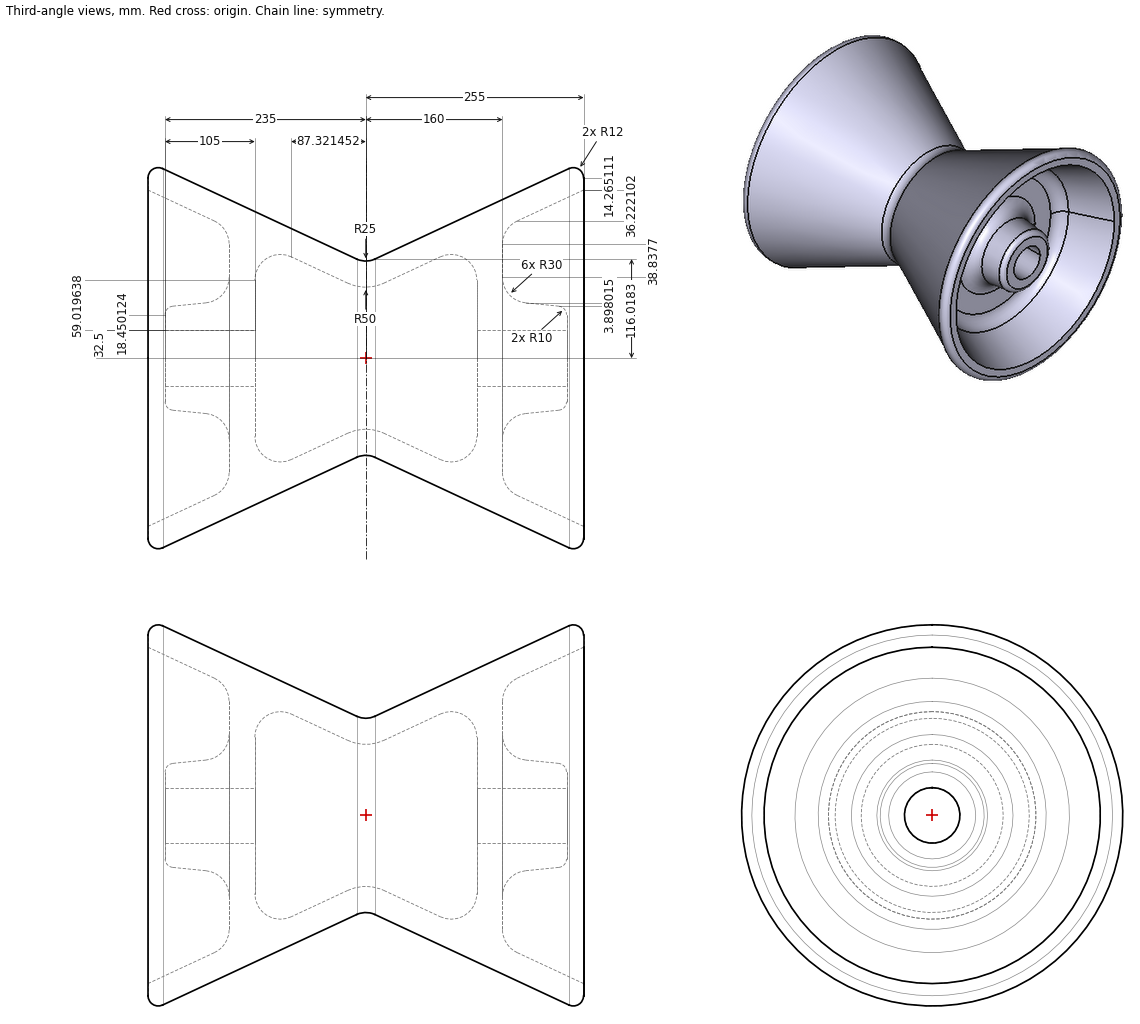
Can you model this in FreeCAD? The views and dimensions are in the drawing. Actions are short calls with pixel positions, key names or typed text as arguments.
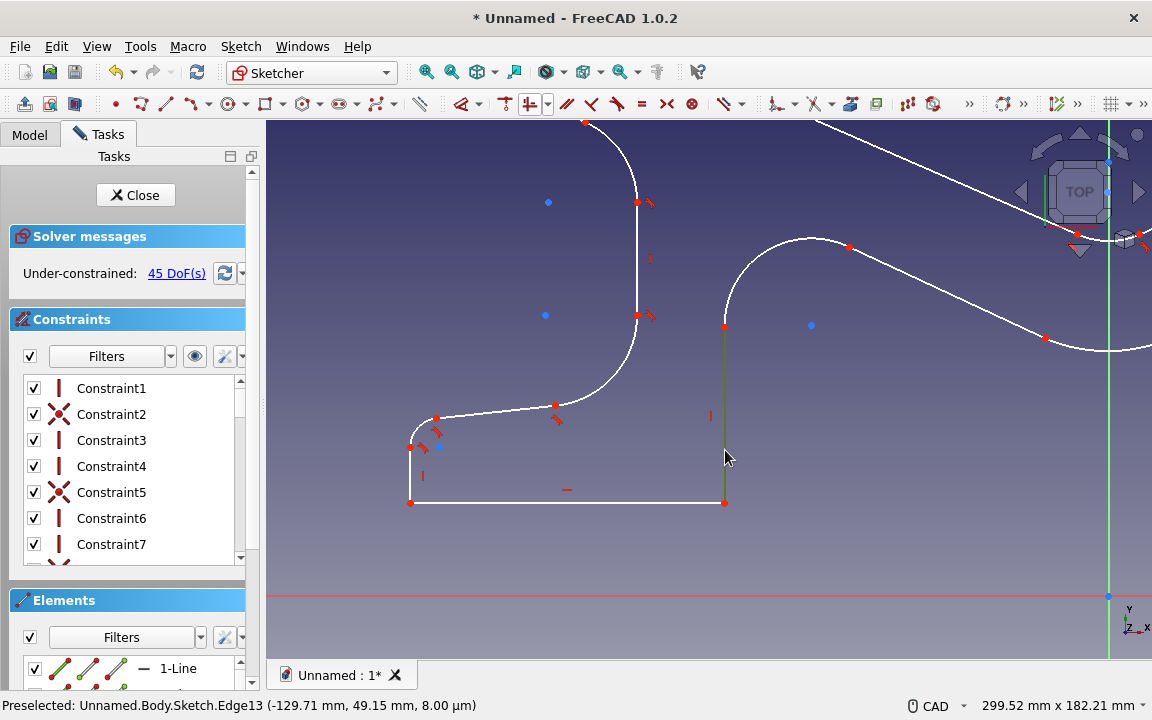
click(798, 240)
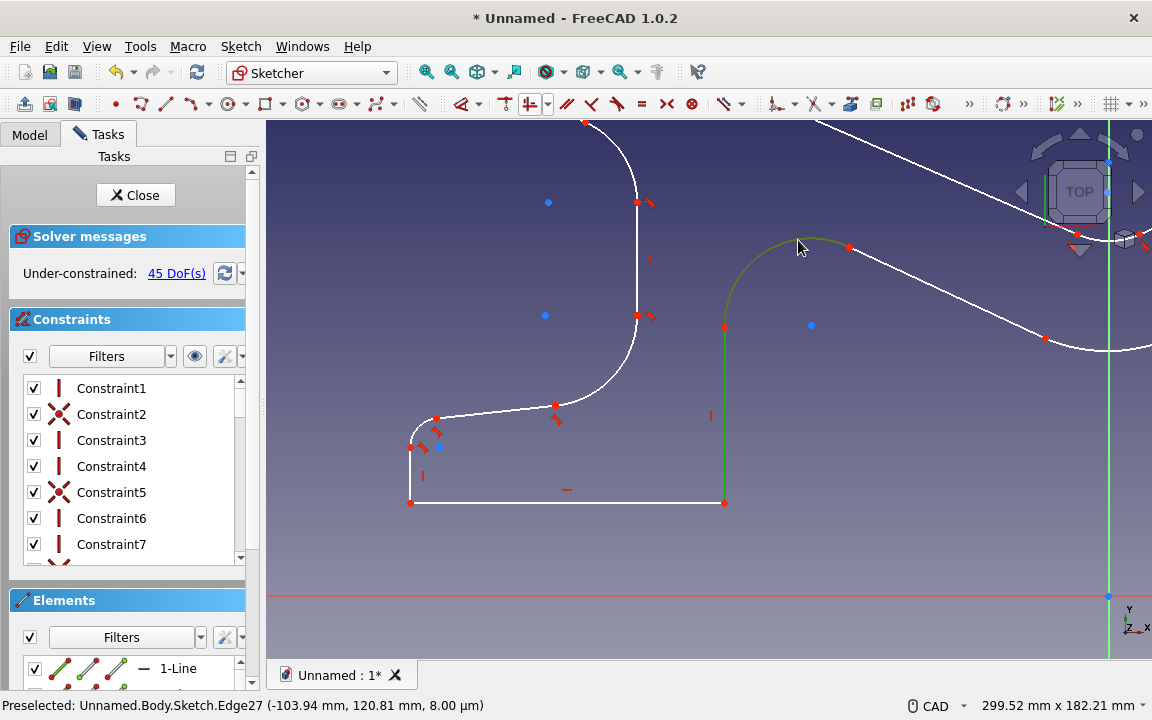
key(t)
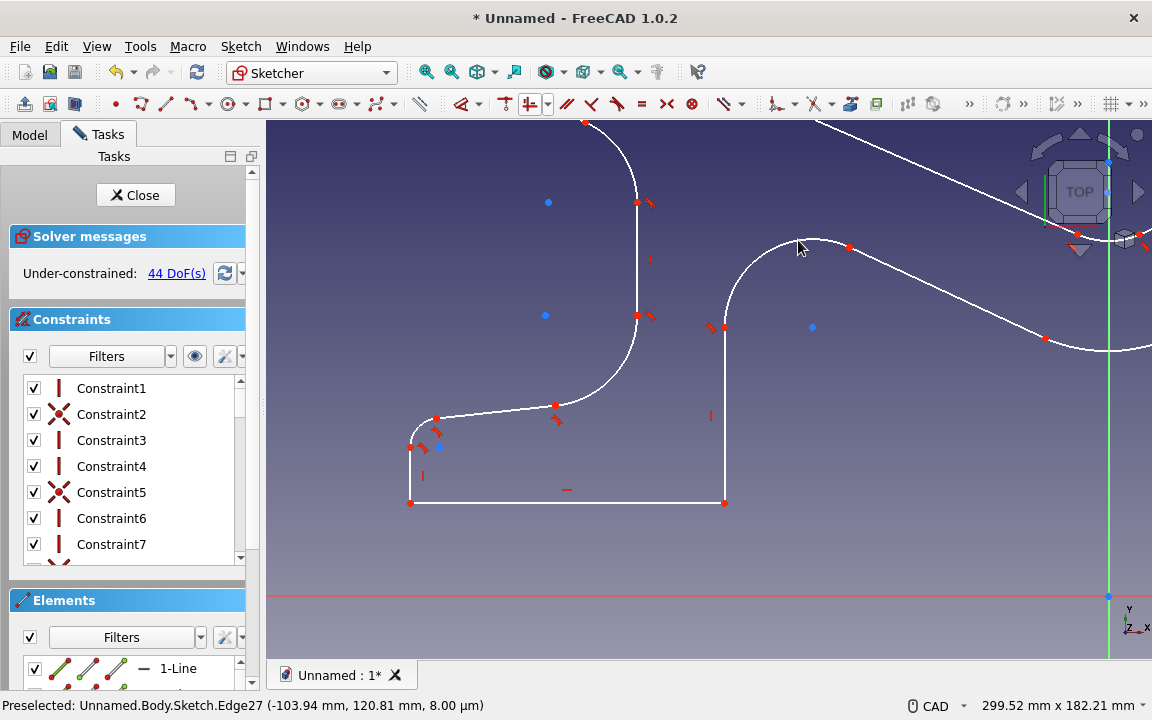
click(908, 275)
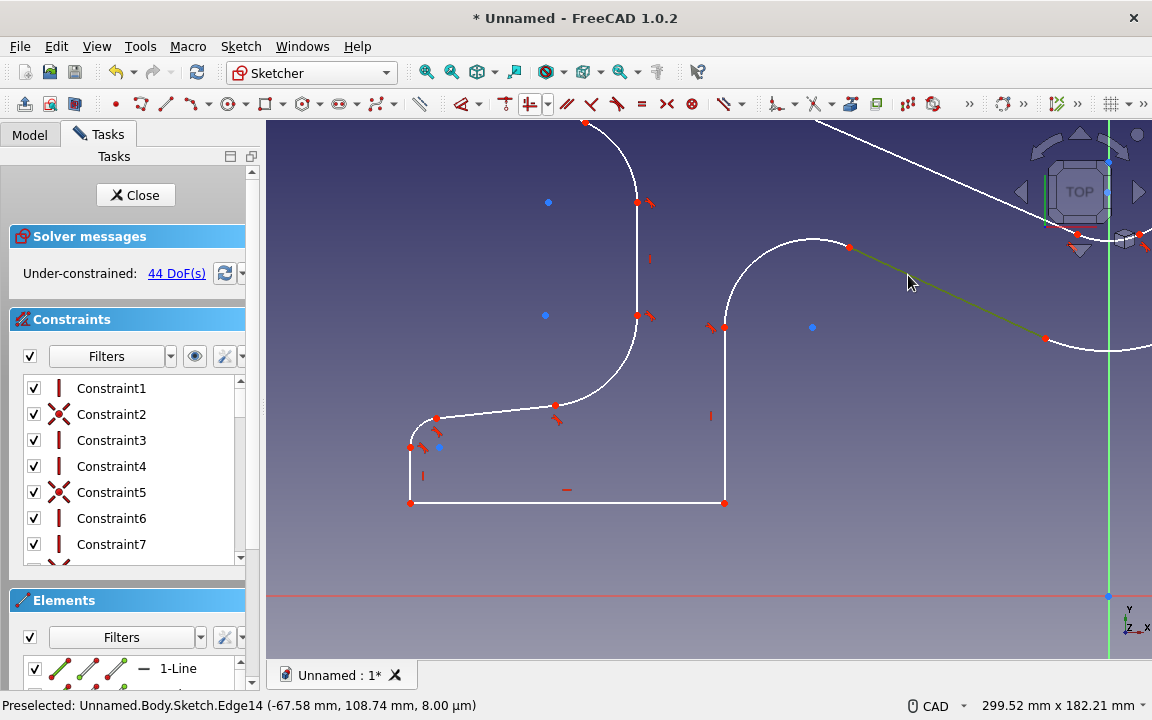
click(798, 241)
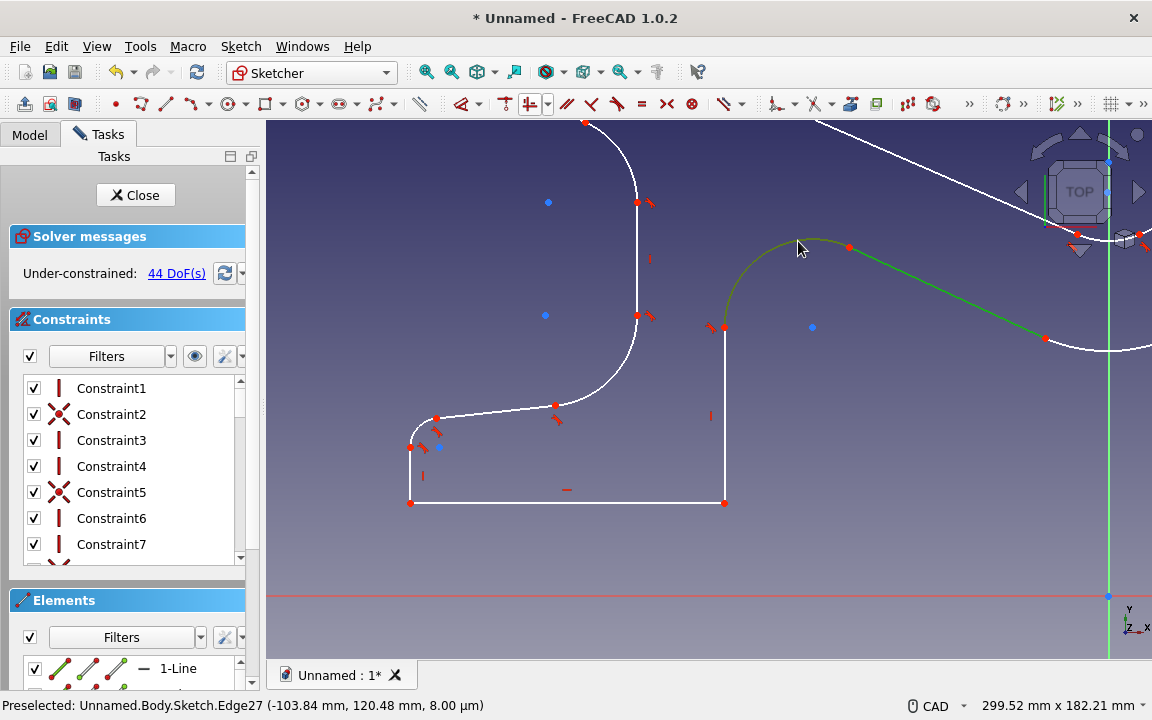
key(t)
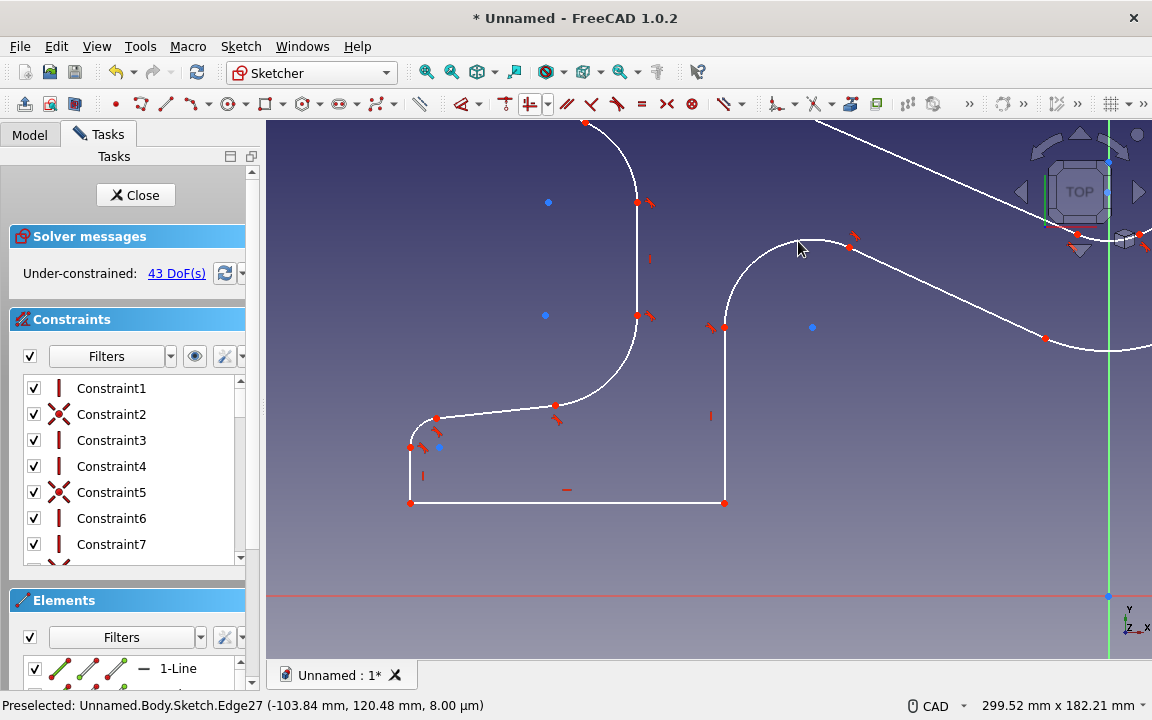
click(908, 275)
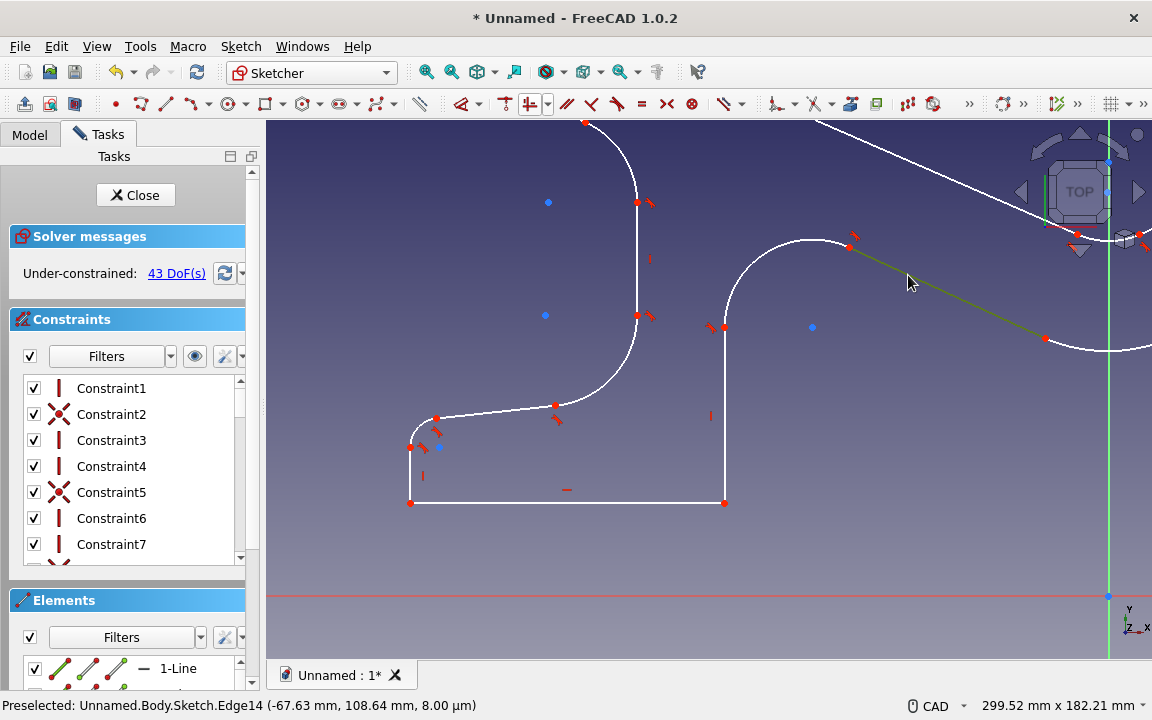
scroll(439, 442, down, 6)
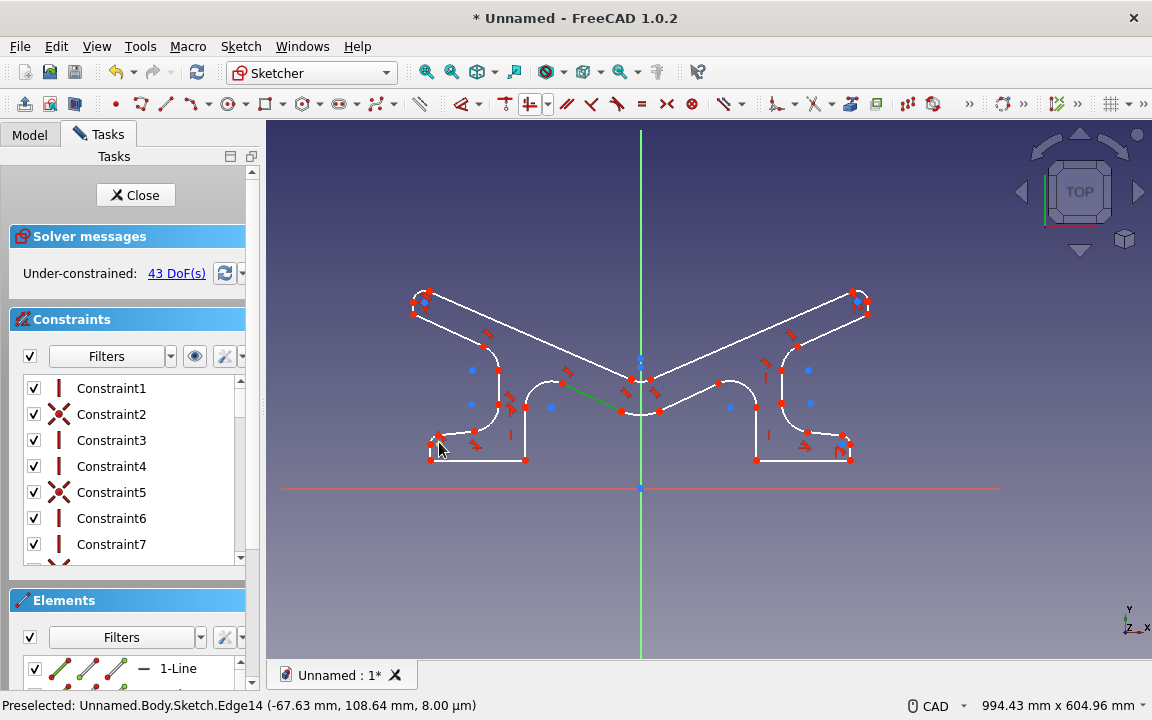
scroll(633, 414, up, 3)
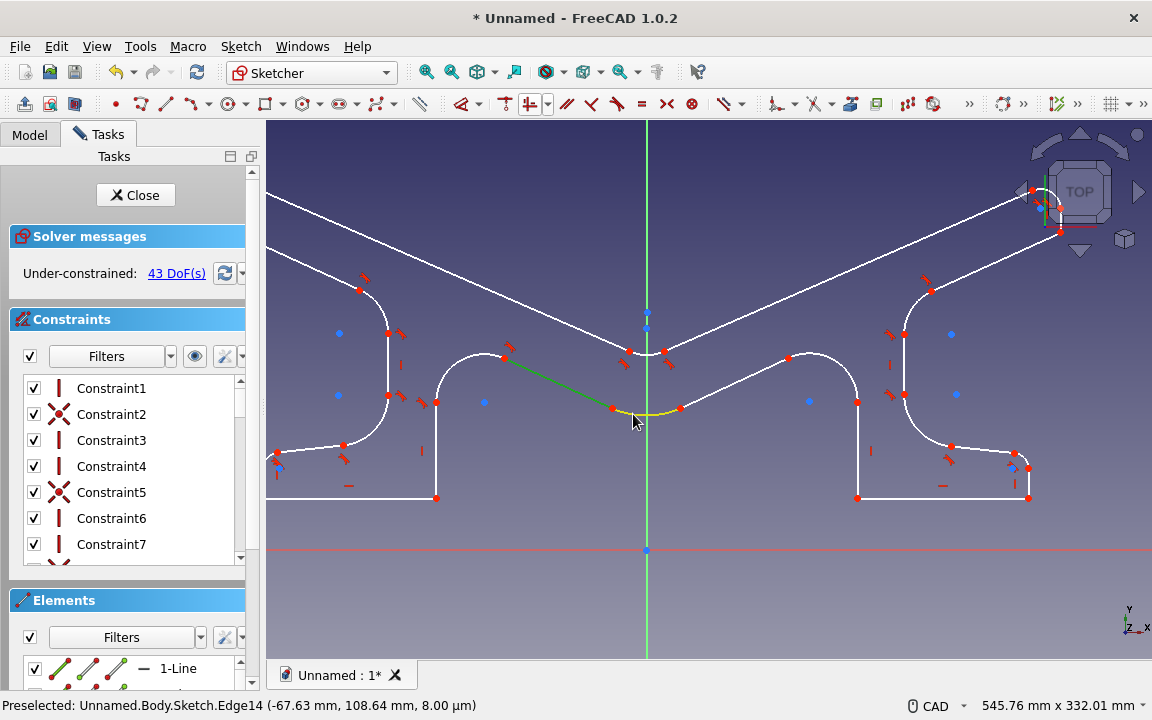
click(632, 414)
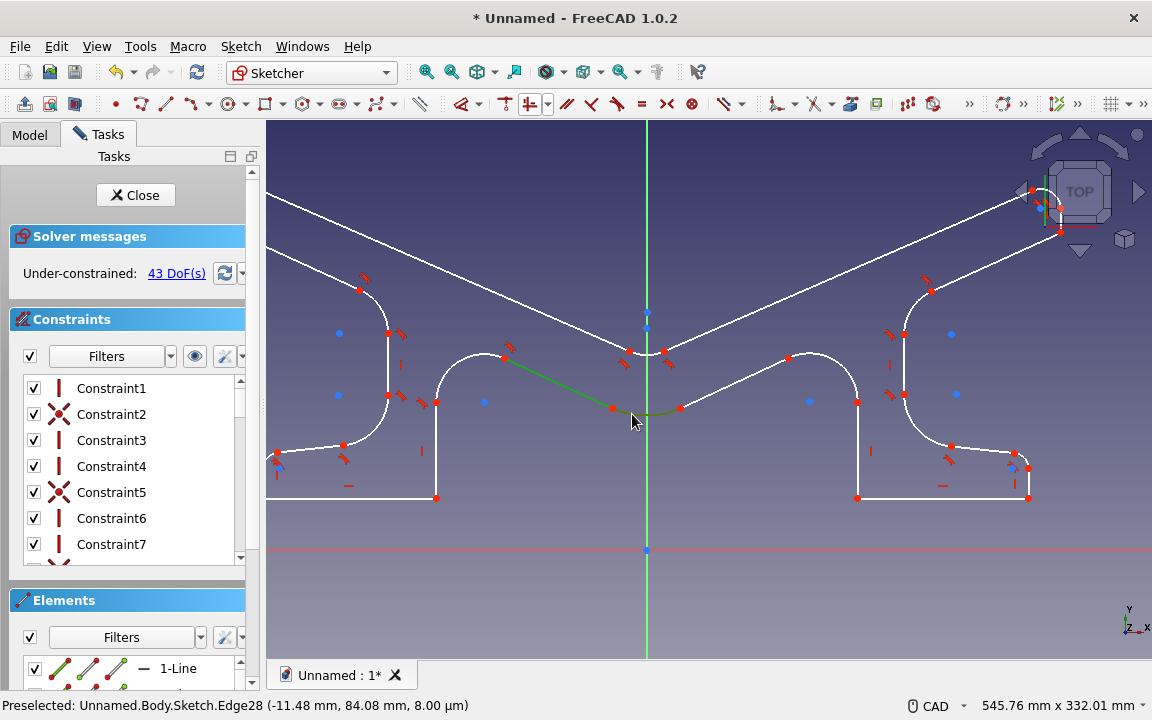
click(617, 104)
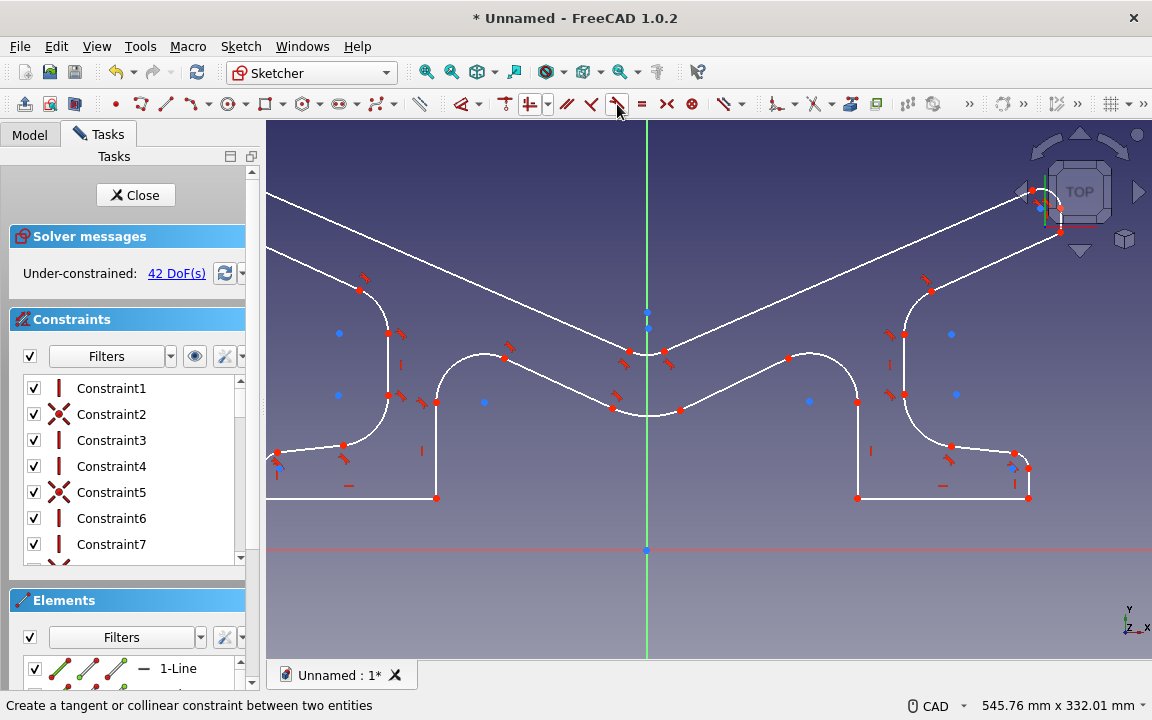
click(713, 395)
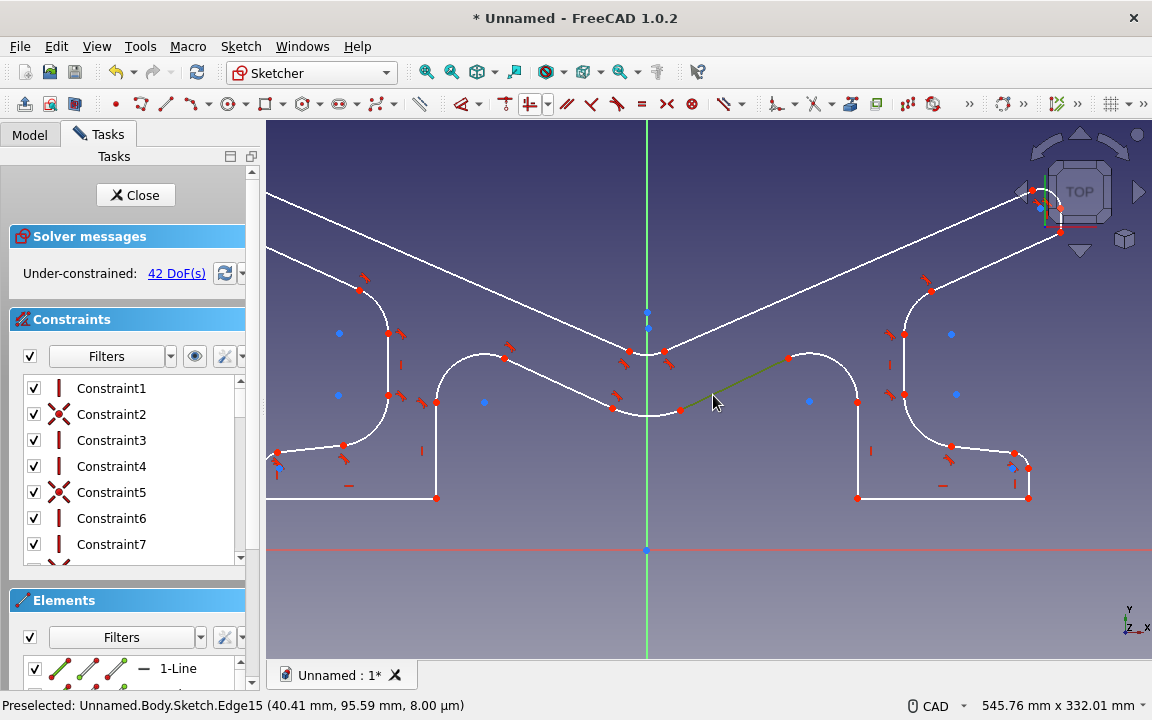
click(632, 415)